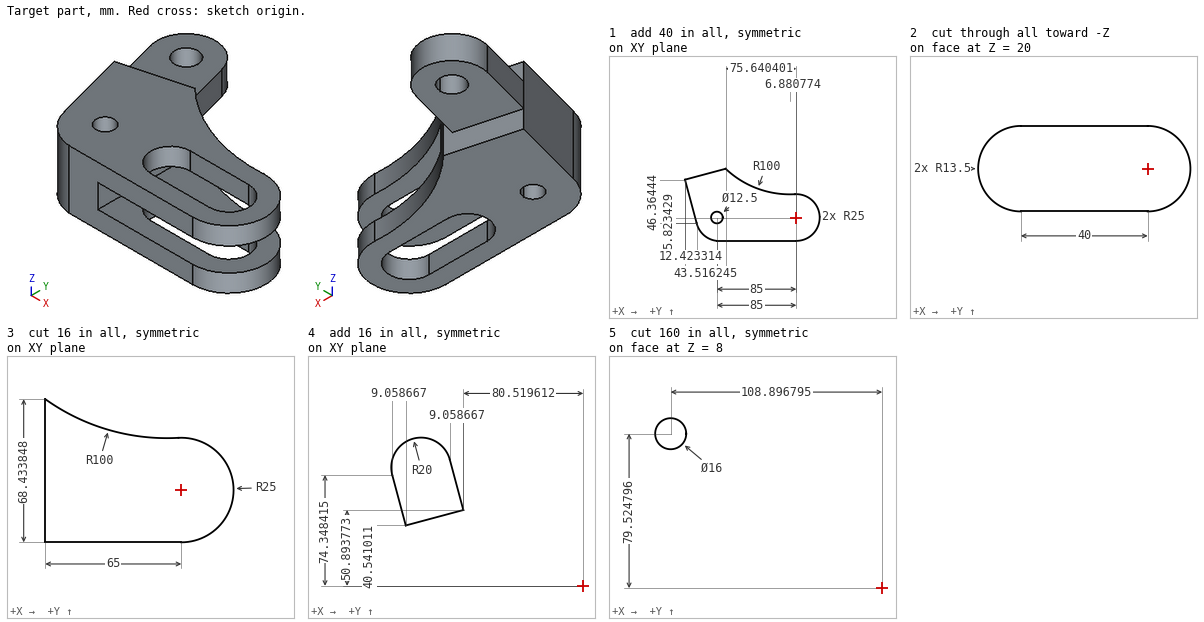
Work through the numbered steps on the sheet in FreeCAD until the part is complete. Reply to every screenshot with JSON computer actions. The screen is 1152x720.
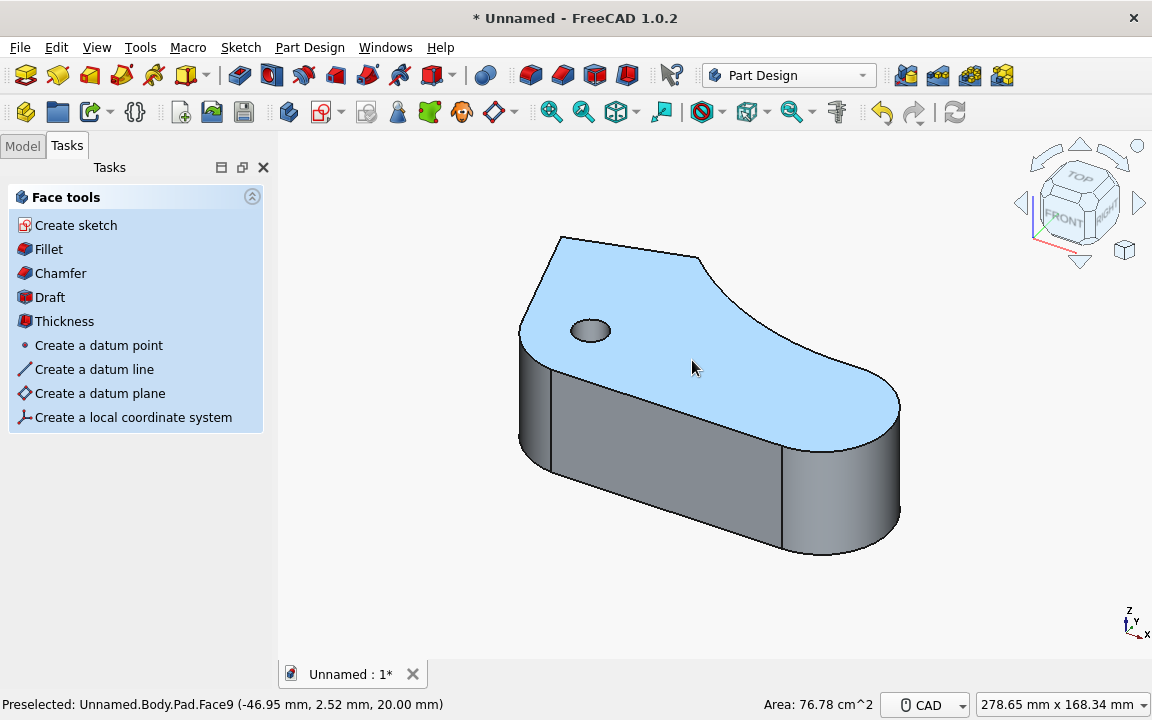
{"action": "left_click", "coordinate": [322, 112]}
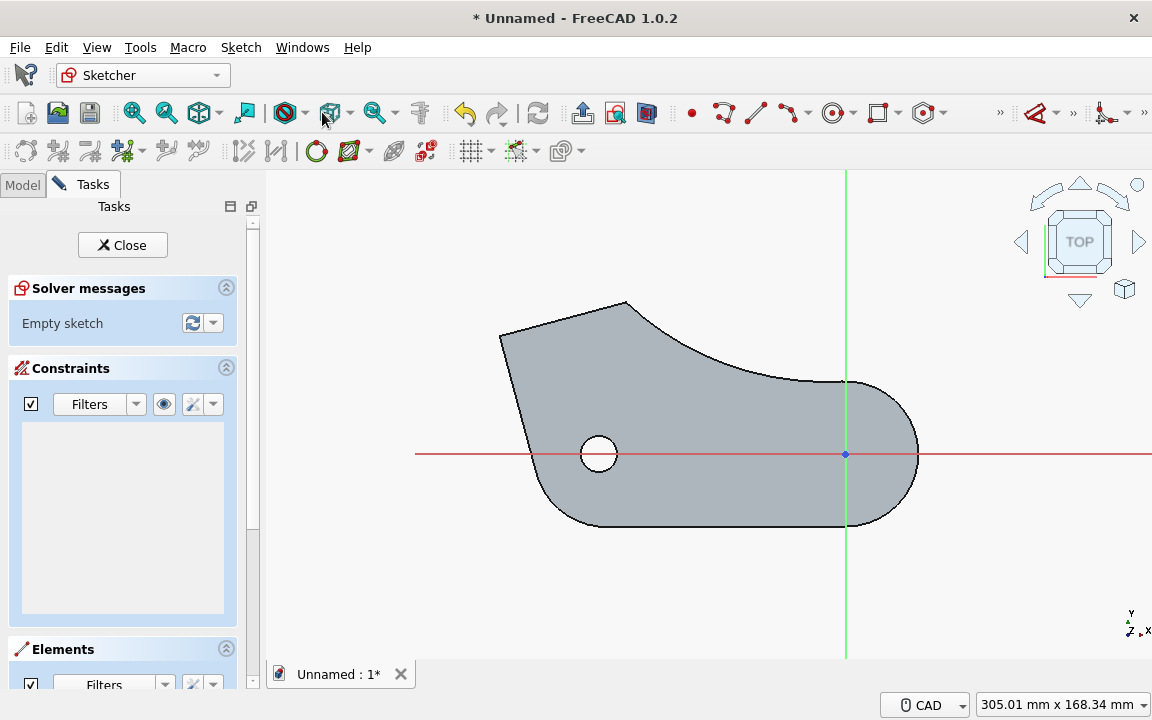
{"action": "scroll", "coordinate": [873, 477], "scroll_direction": "up", "scroll_amount": 5}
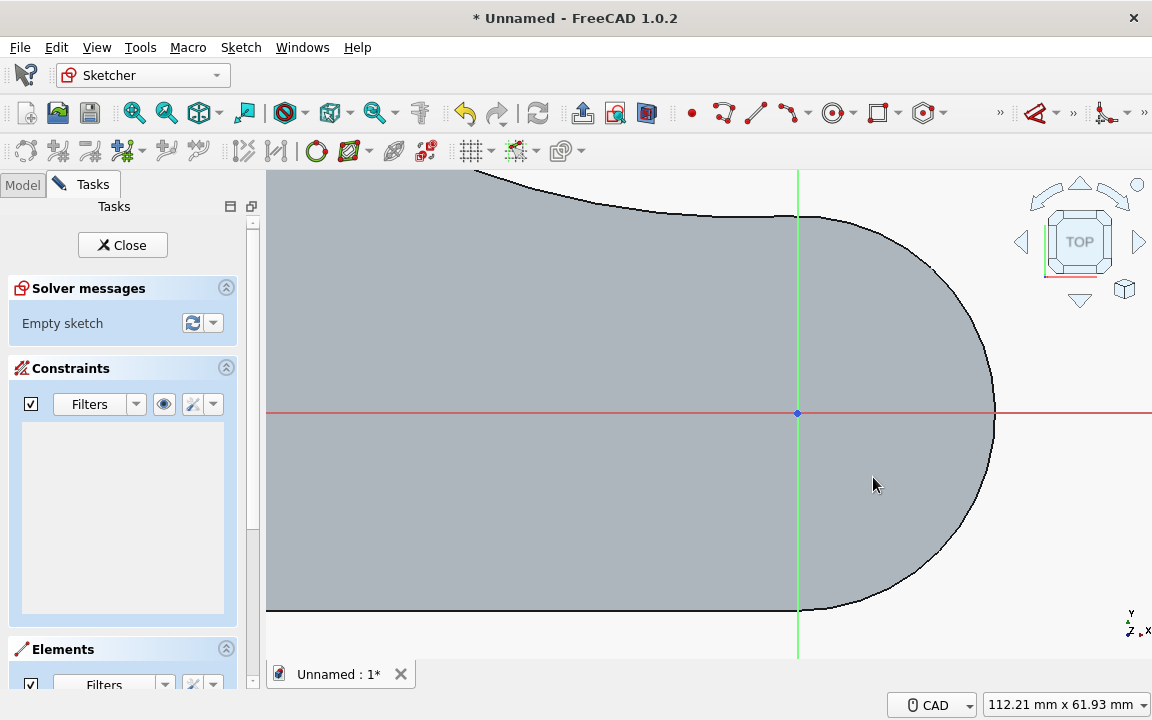
{"action": "key", "text": "g s"}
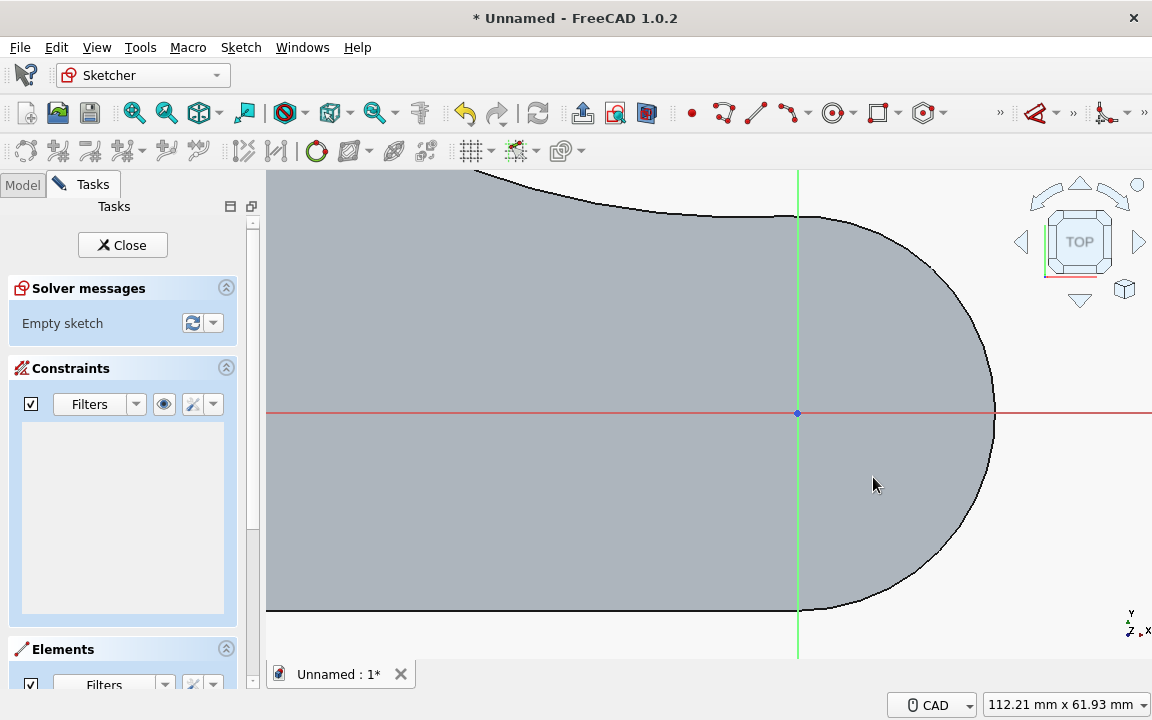
{"action": "left_click", "coordinate": [798, 413]}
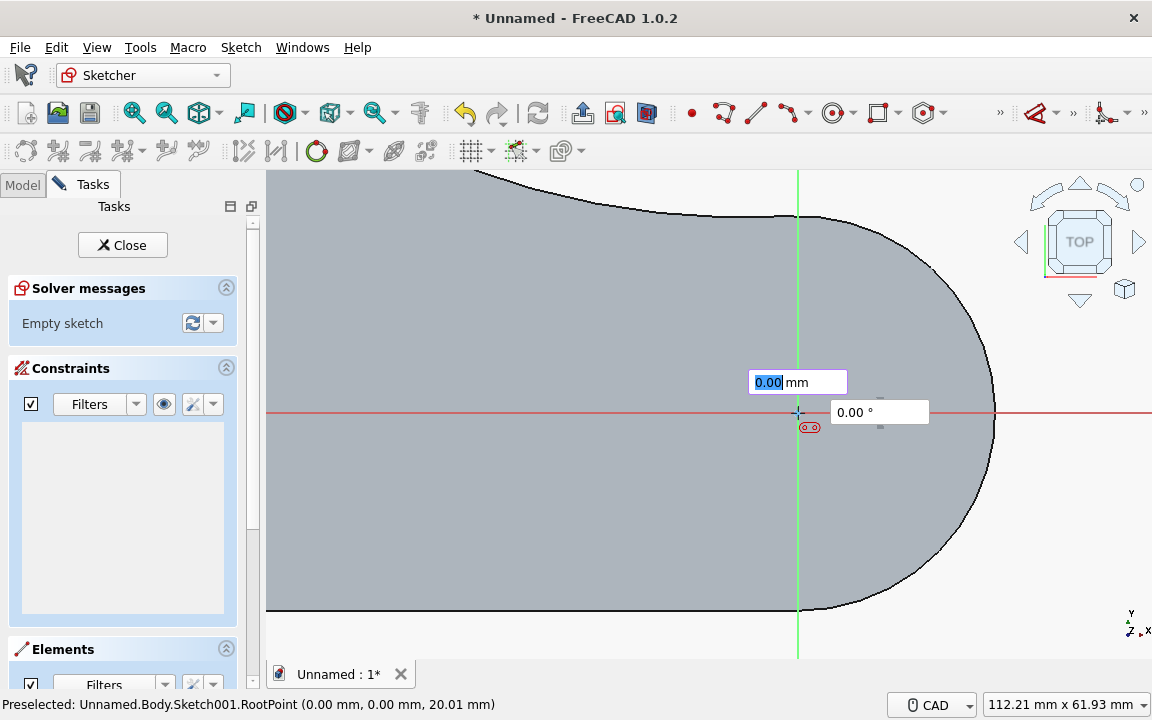
{"action": "left_click", "coordinate": [482, 404]}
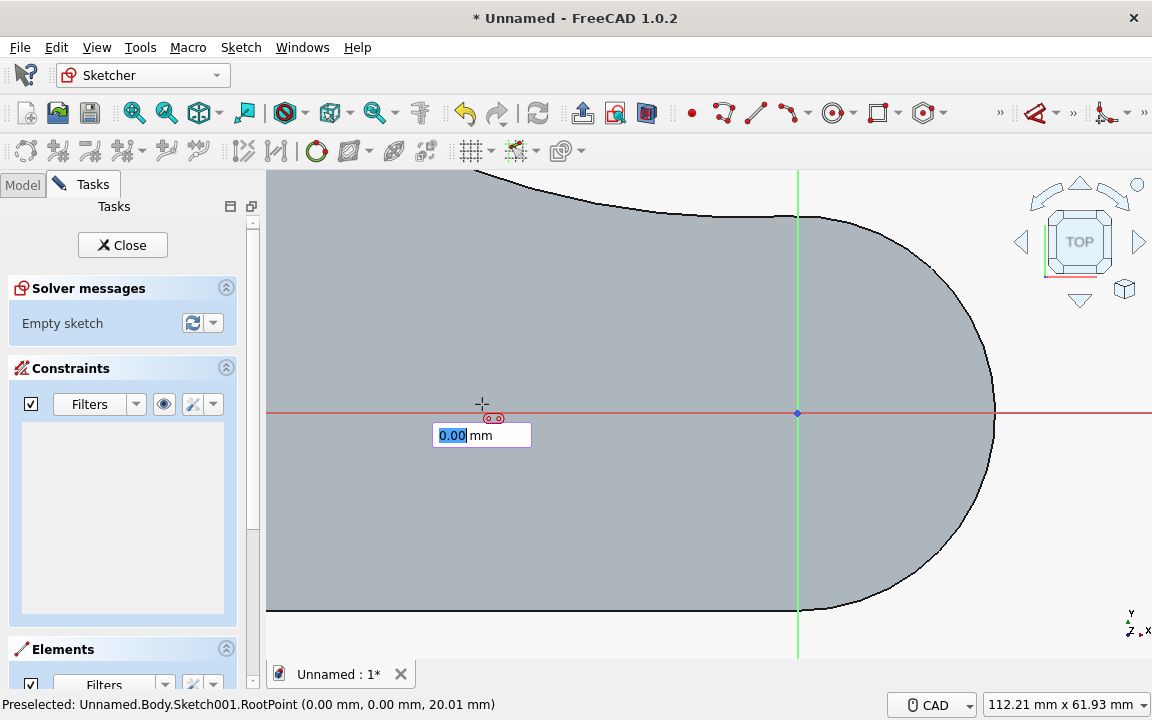
{"action": "left_click", "coordinate": [640, 307]}
{"action": "key", "text": "Escape"}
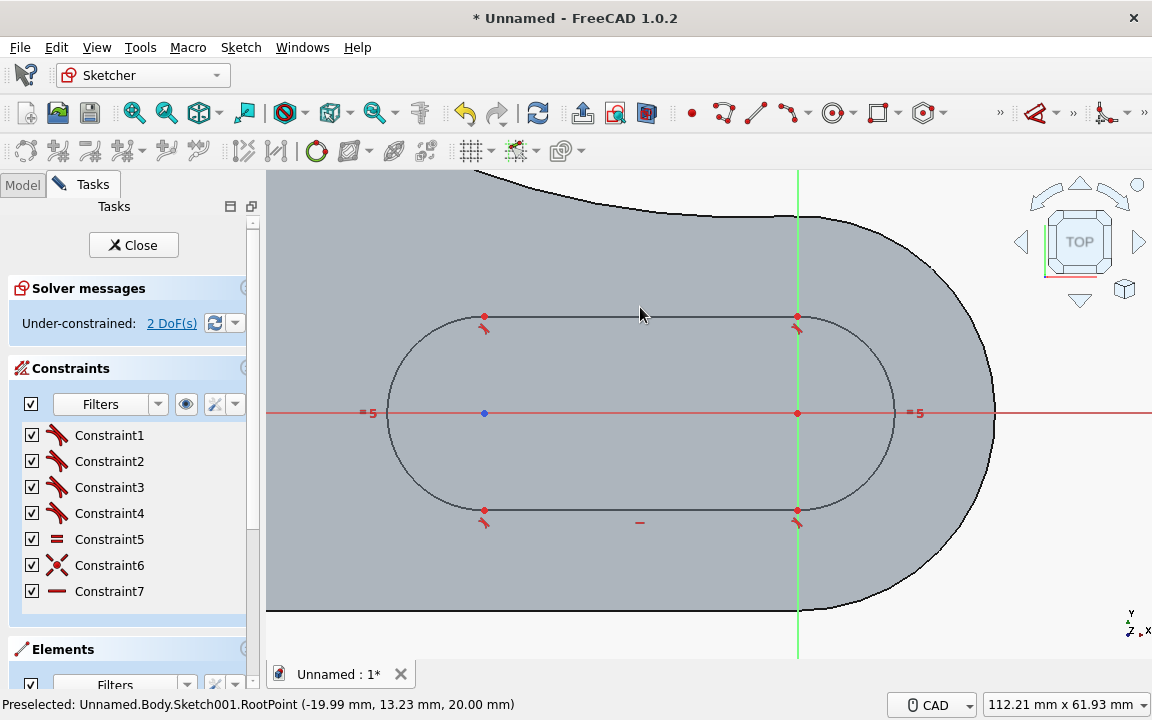
{"action": "left_click", "coordinate": [1036, 114]}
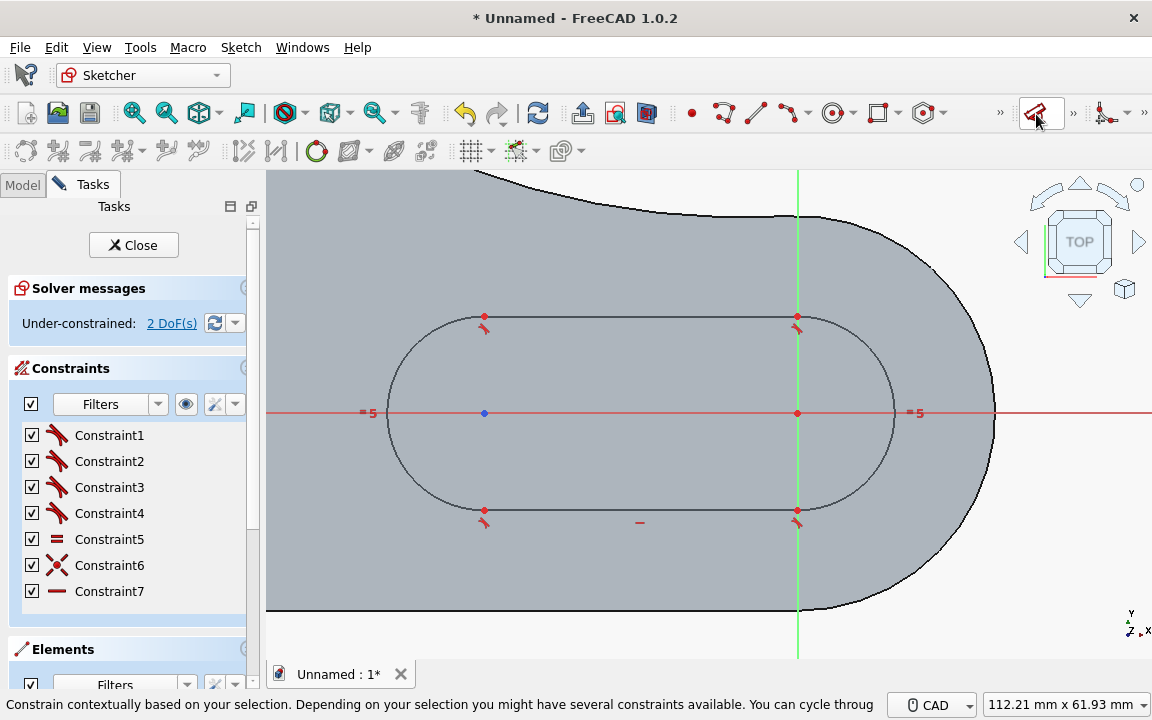
{"action": "left_click", "coordinate": [876, 470]}
{"action": "left_click", "coordinate": [902, 489]}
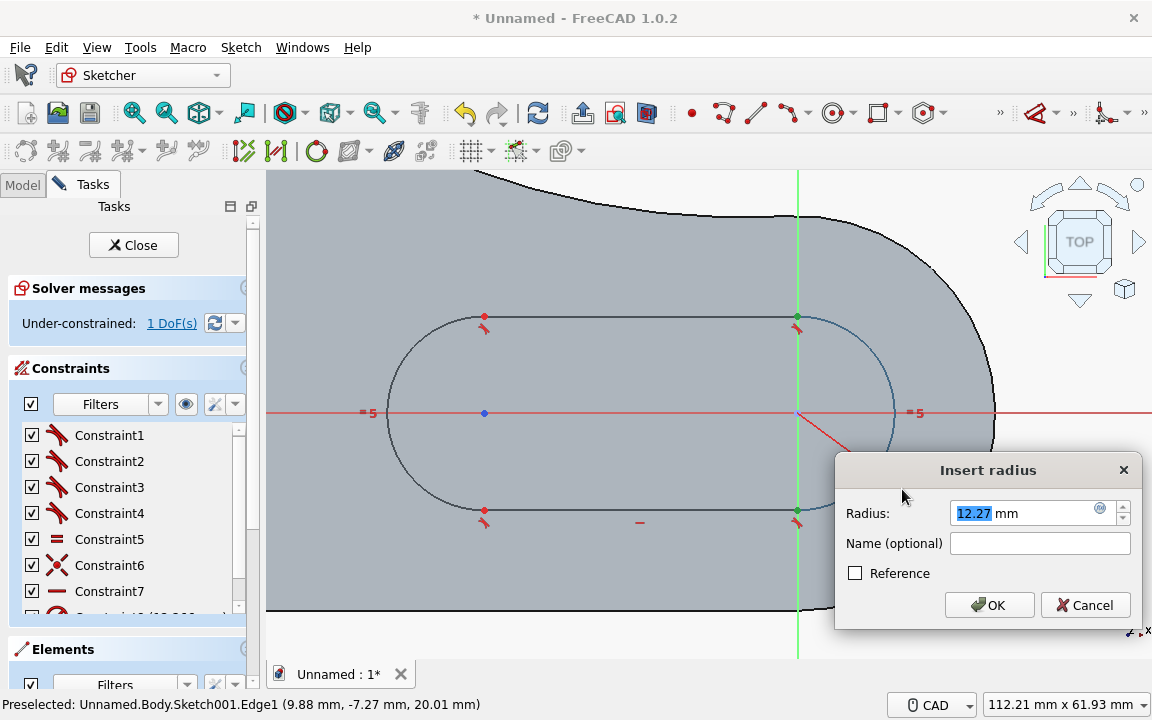
{"action": "type", "text": "13.5"}
{"action": "key", "text": "Return"}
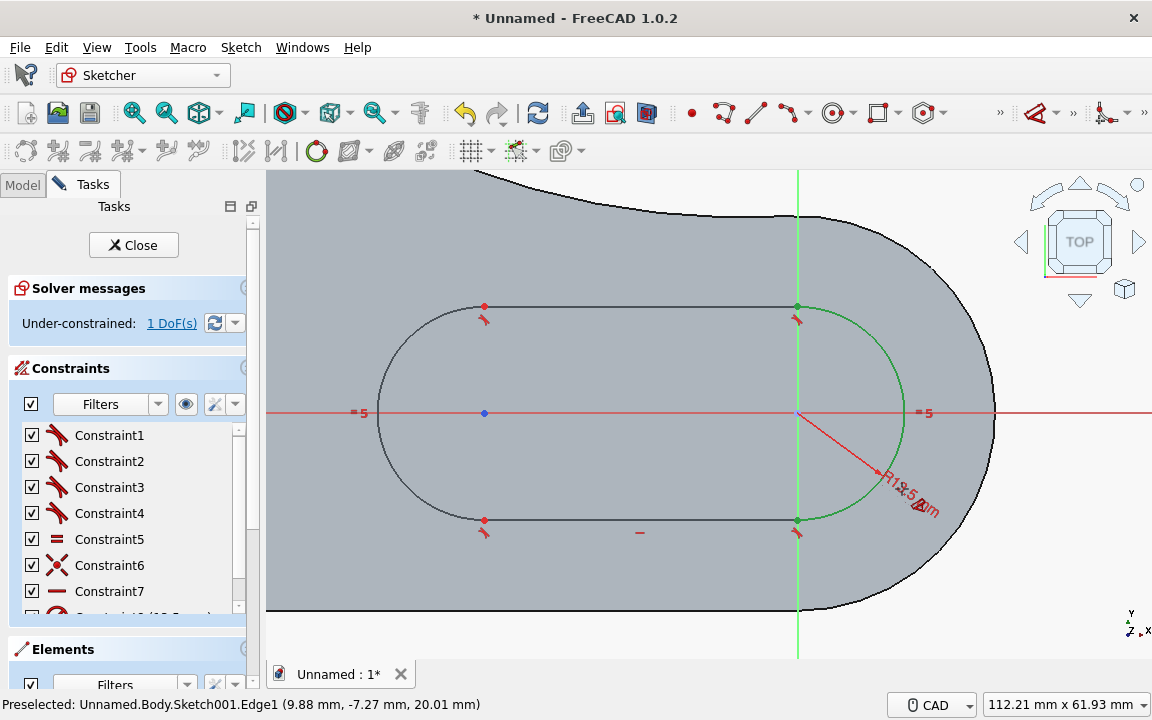
{"action": "left_click", "coordinate": [704, 520]}
{"action": "left_click", "coordinate": [641, 554]}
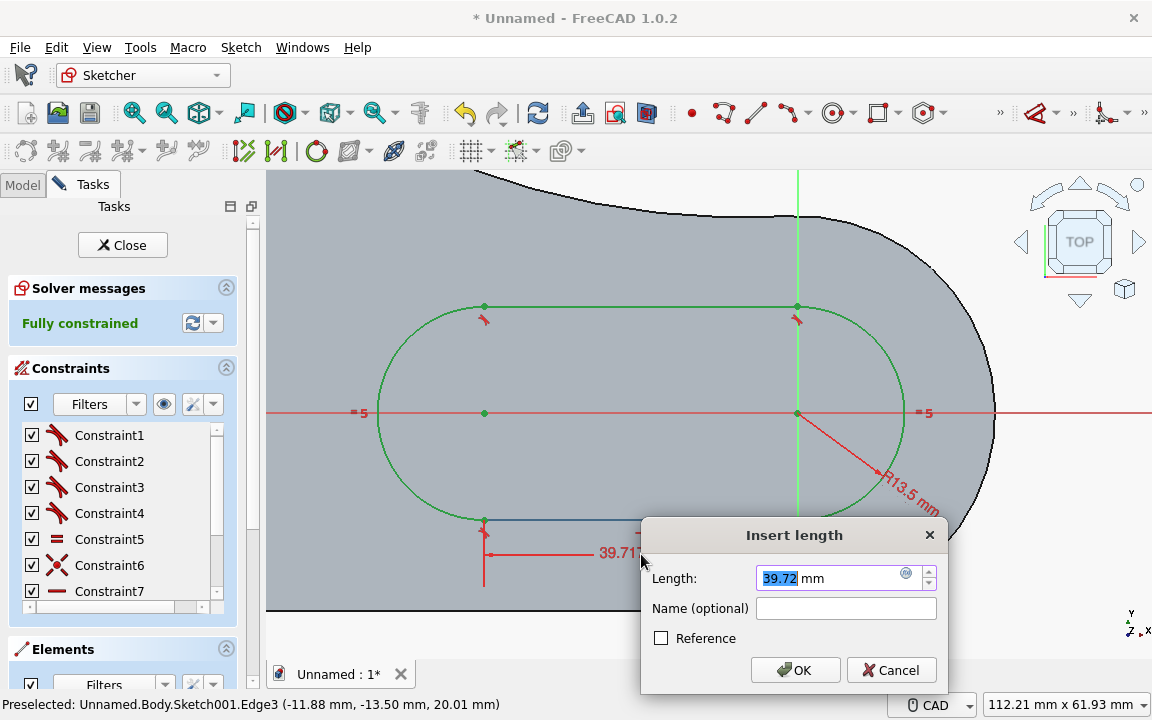
{"action": "type", "text": "40"}
{"action": "key", "text": "Return"}
{"action": "key", "text": "Escape"}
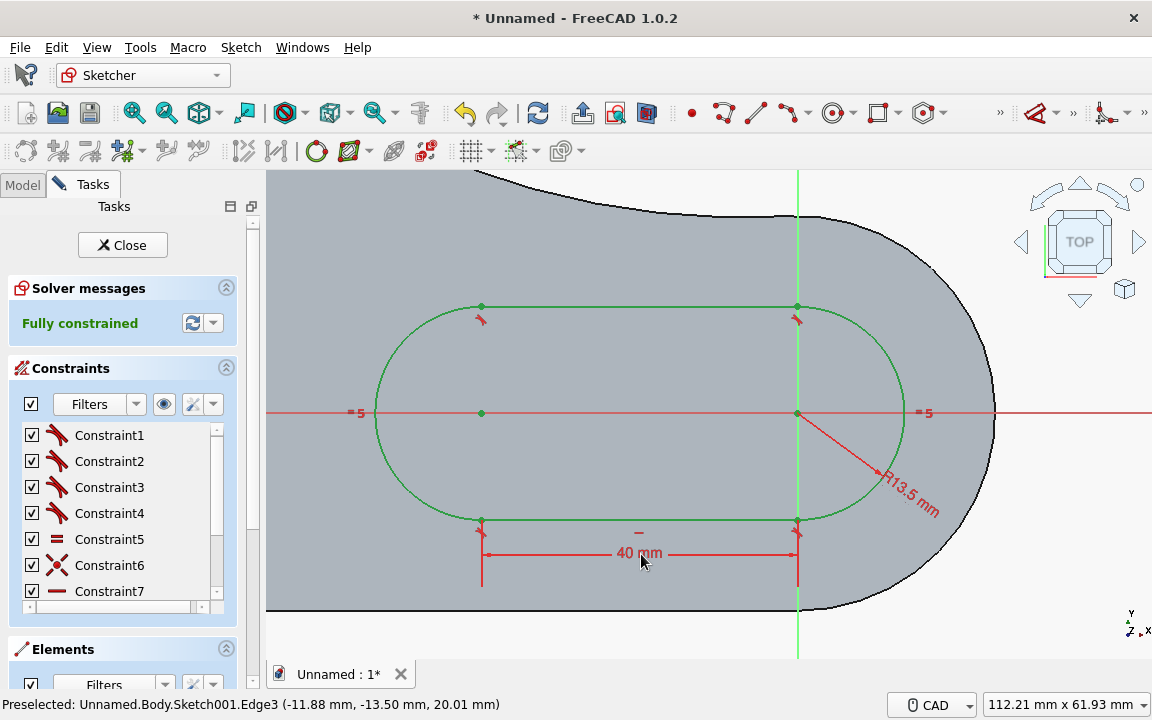
{"action": "left_click", "coordinate": [123, 245]}